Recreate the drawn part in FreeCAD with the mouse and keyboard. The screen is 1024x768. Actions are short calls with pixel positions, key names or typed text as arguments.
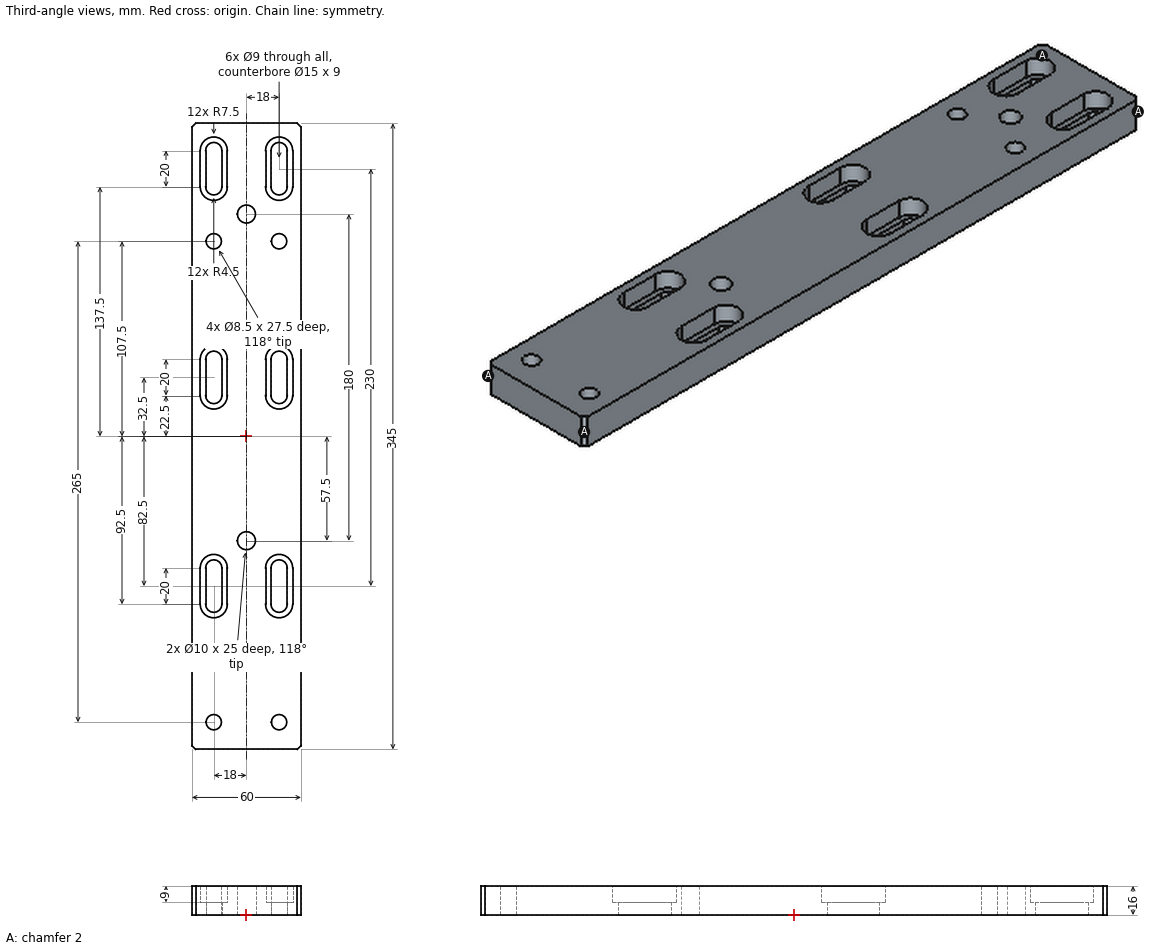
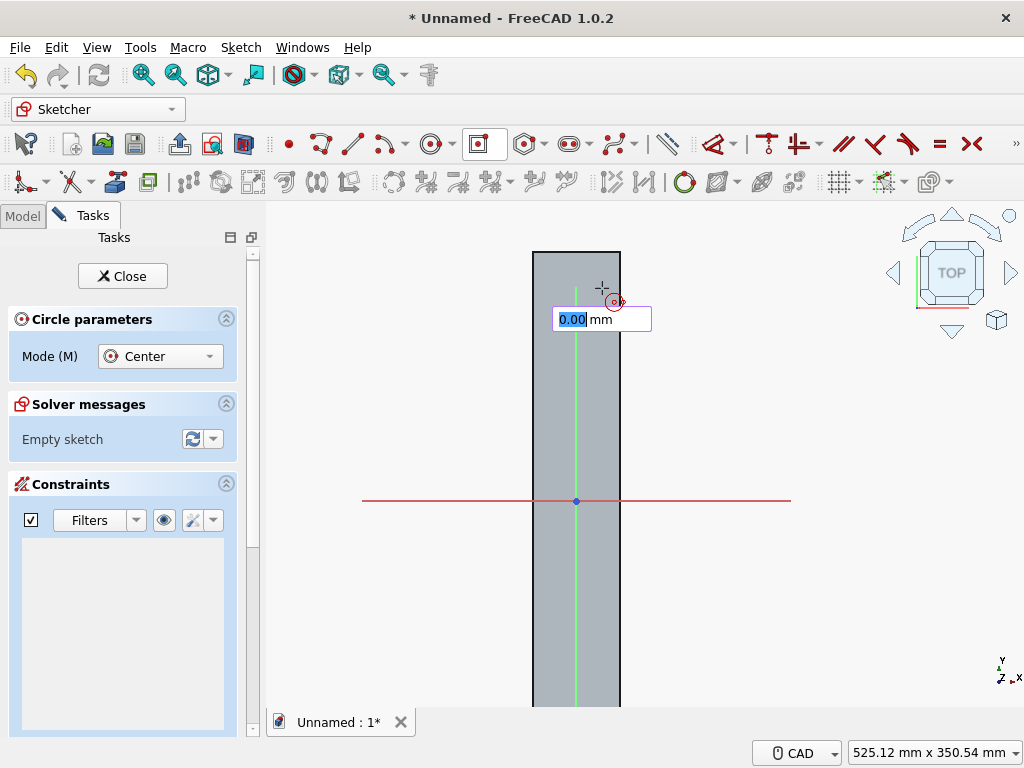
scroll(607, 283, up, 5)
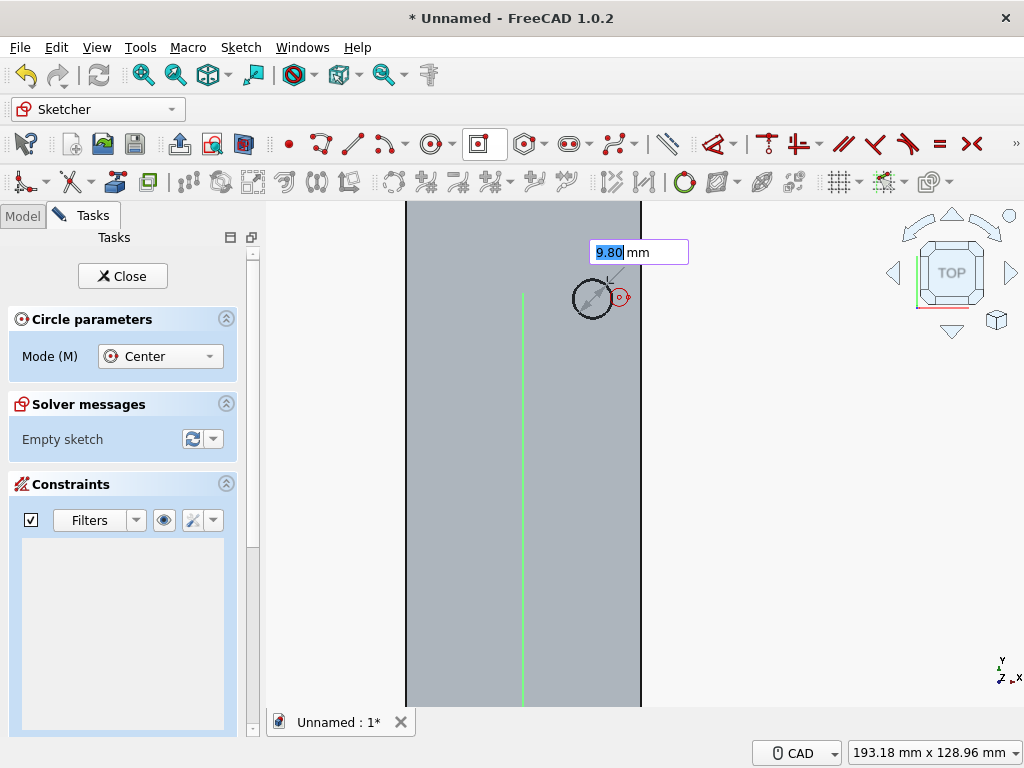
click(606, 284)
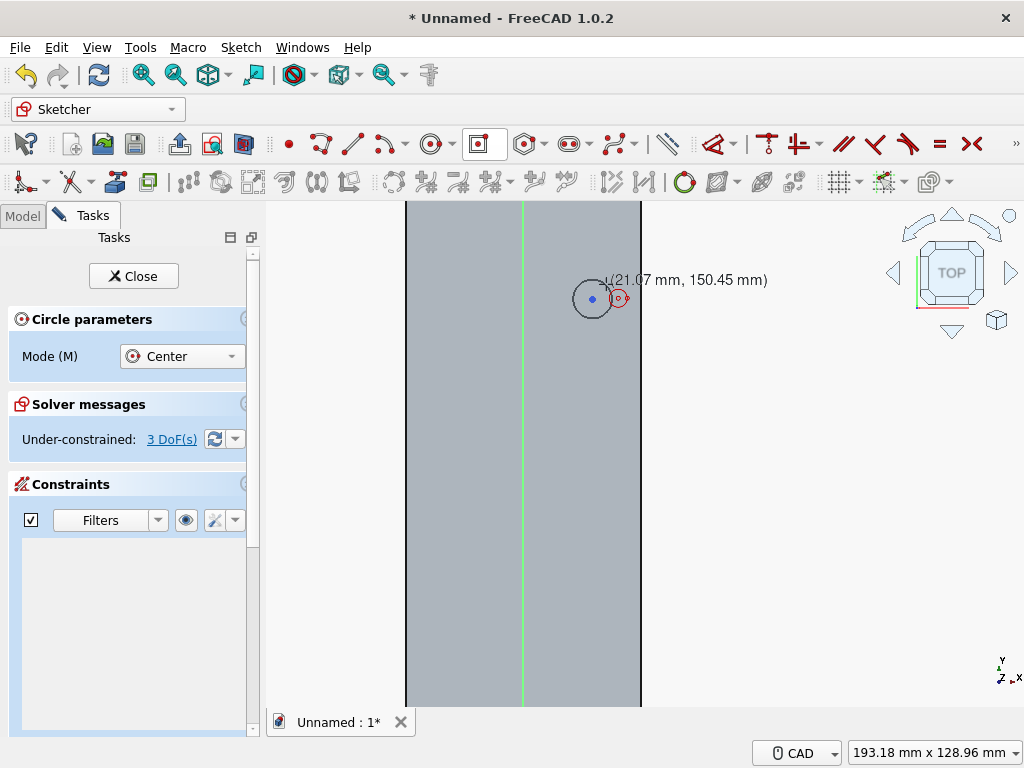
scroll(607, 283, down, 5)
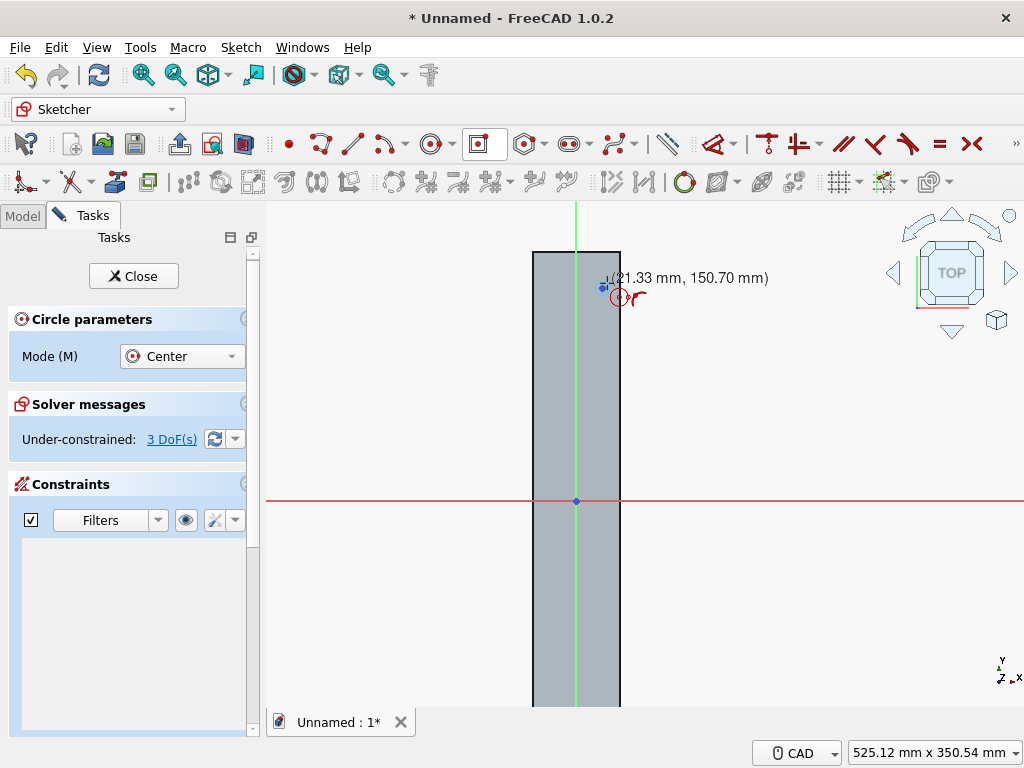
scroll(551, 620, up, 7)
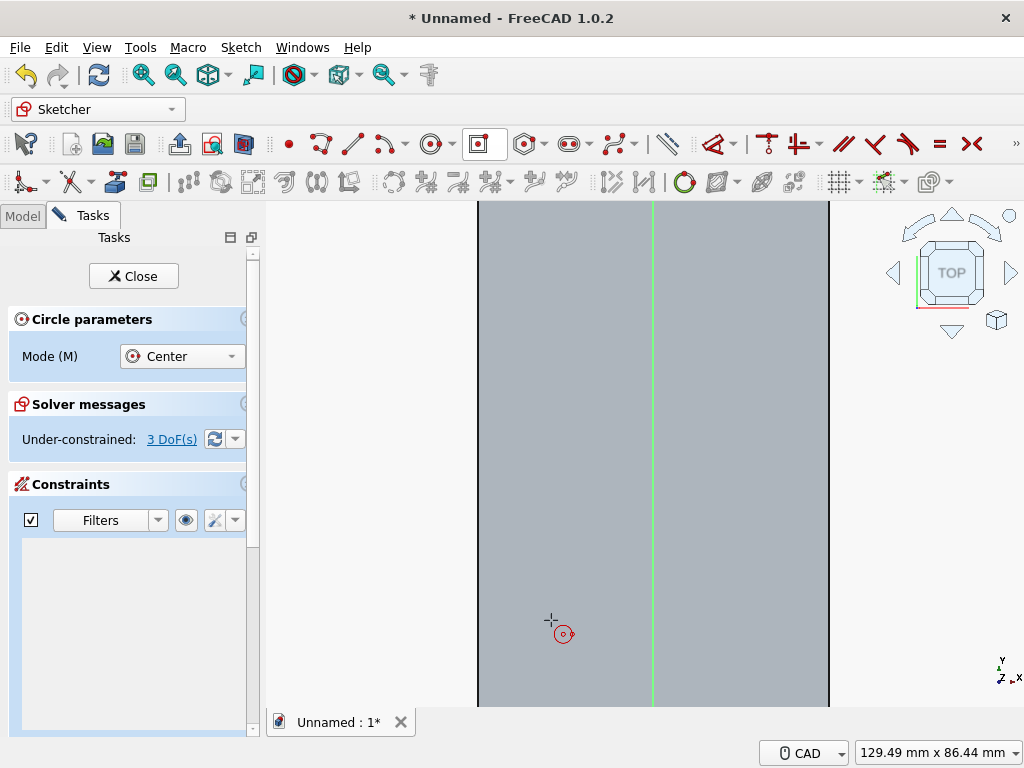
scroll(551, 621, down, 7)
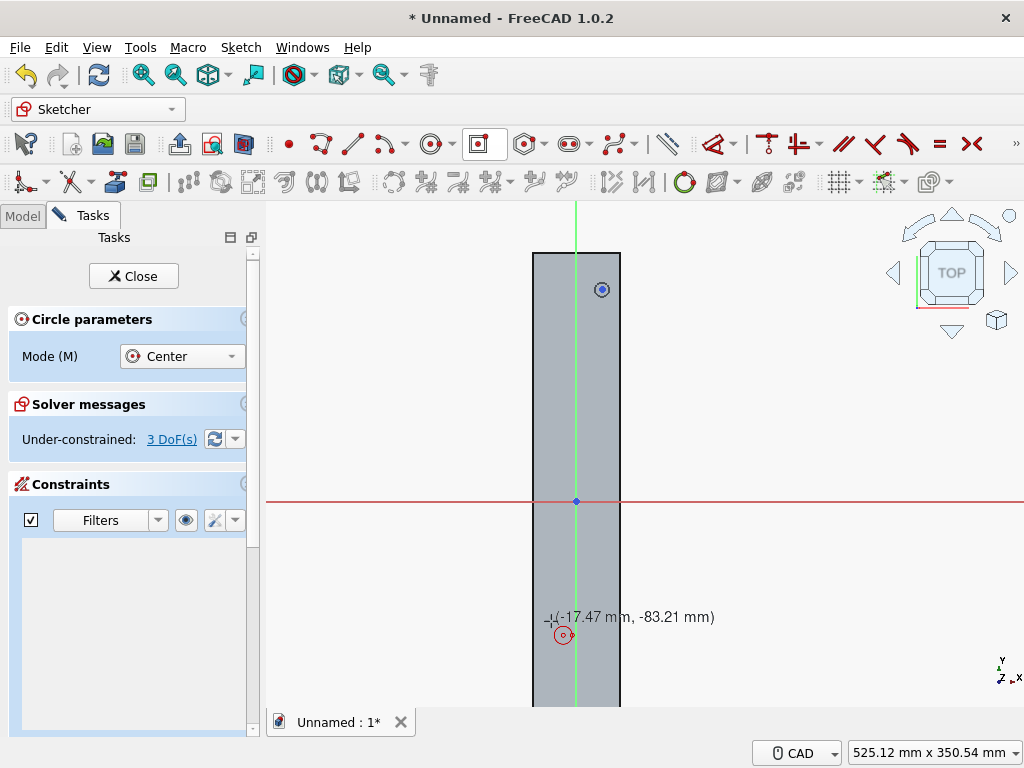
click(551, 621)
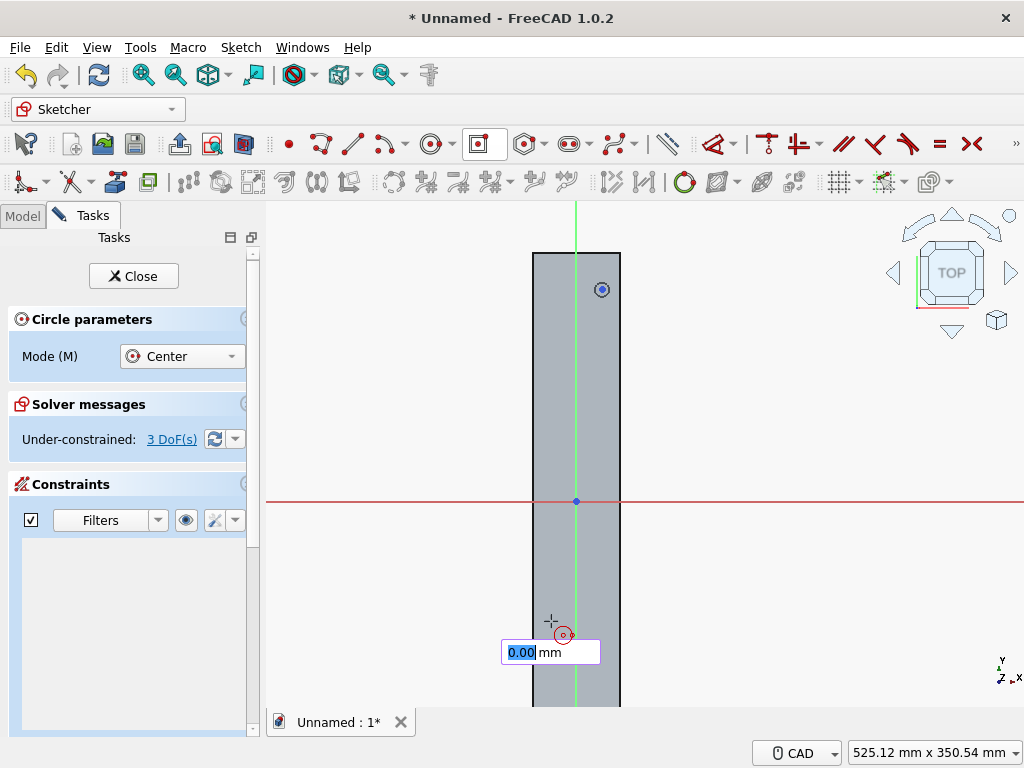
scroll(555, 616, up, 5)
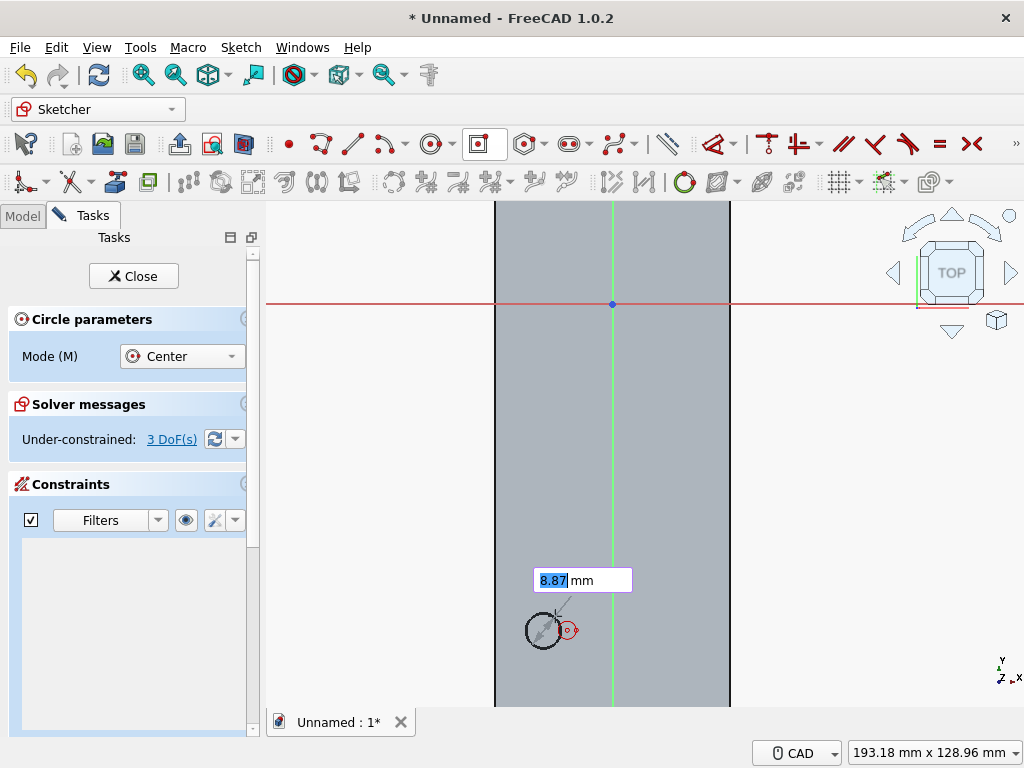
click(555, 615)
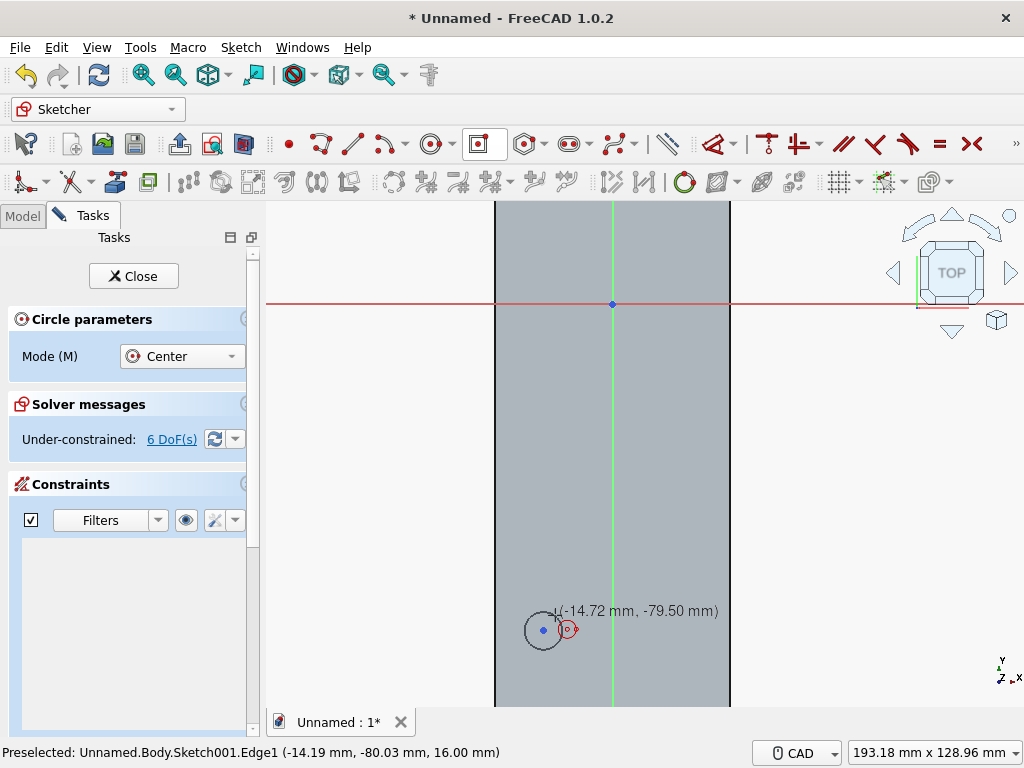
scroll(555, 615, down, 5)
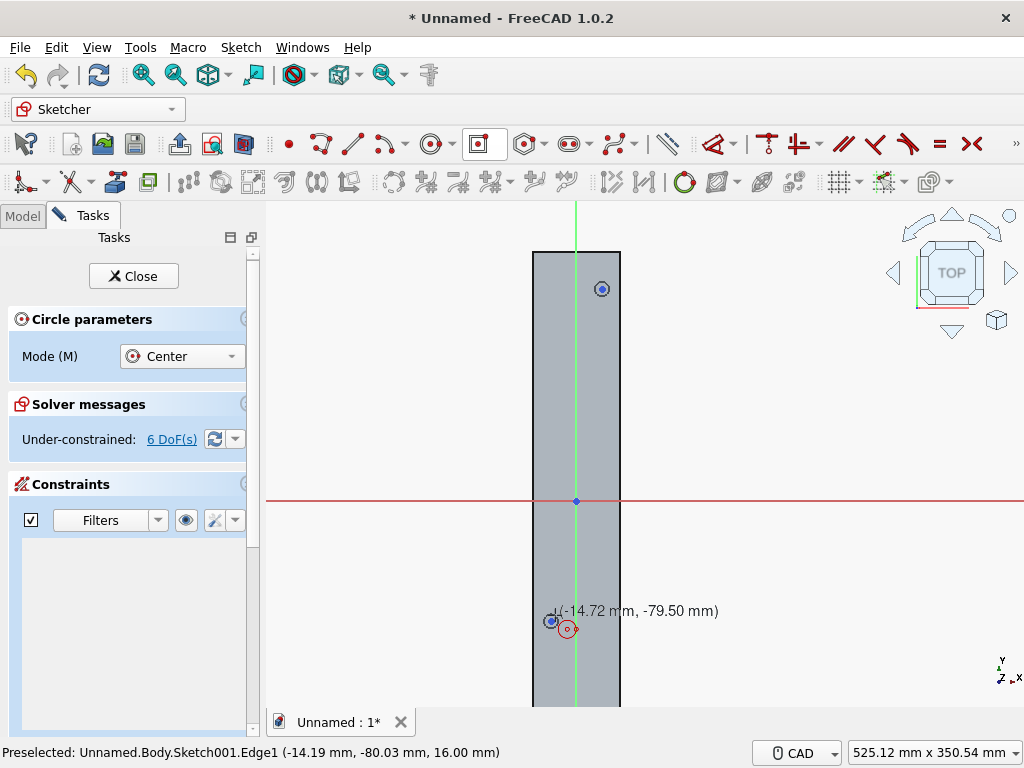
scroll(551, 288, up, 7)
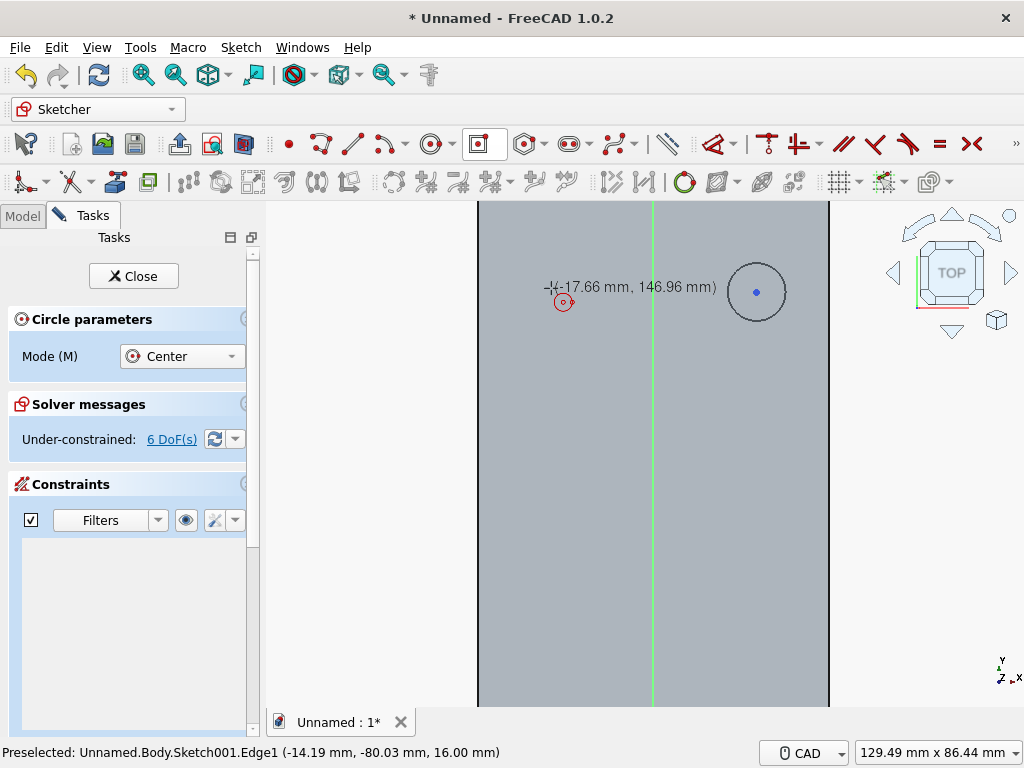
scroll(551, 288, down, 7)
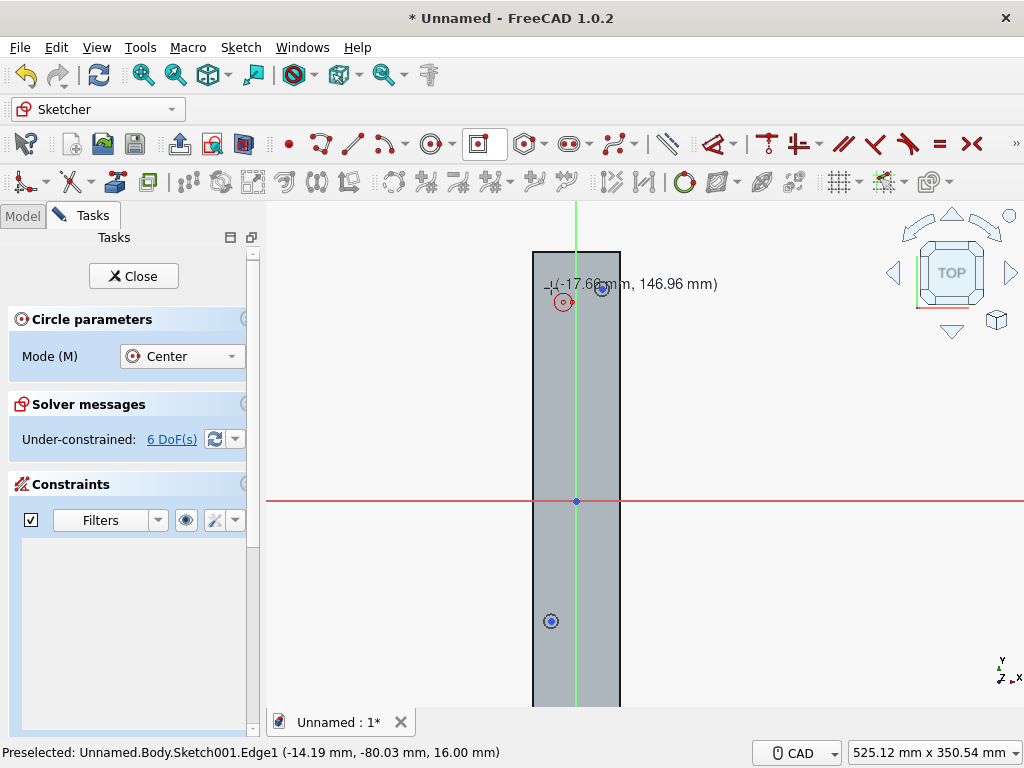
click(551, 288)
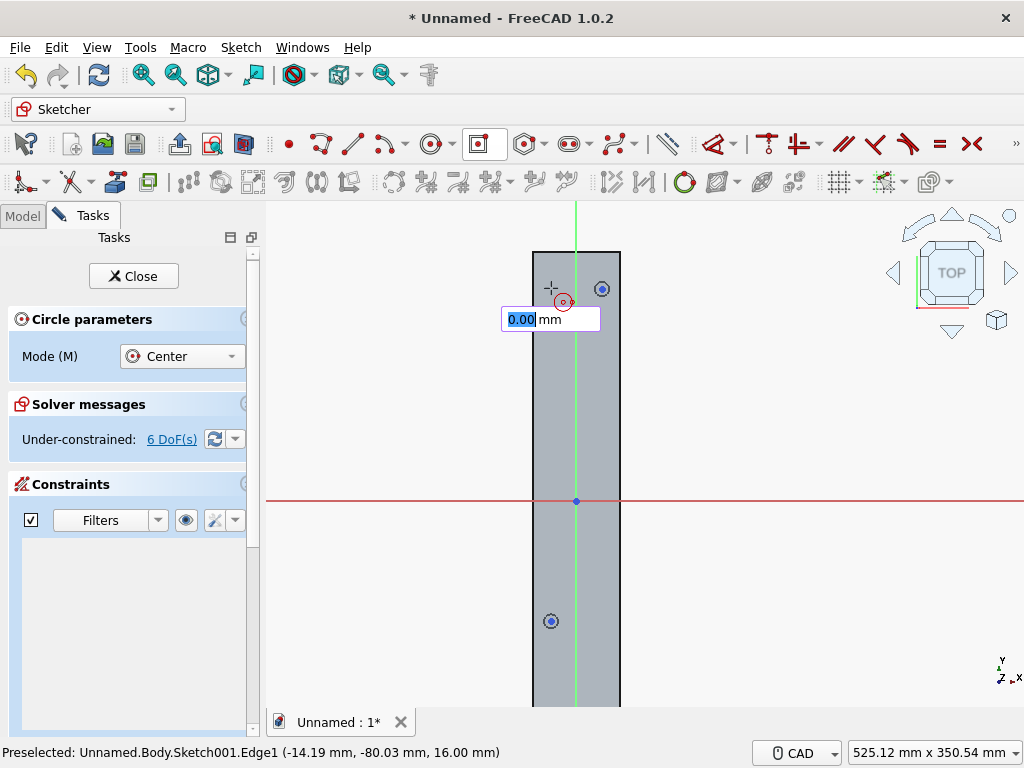
scroll(555, 284, up, 5)